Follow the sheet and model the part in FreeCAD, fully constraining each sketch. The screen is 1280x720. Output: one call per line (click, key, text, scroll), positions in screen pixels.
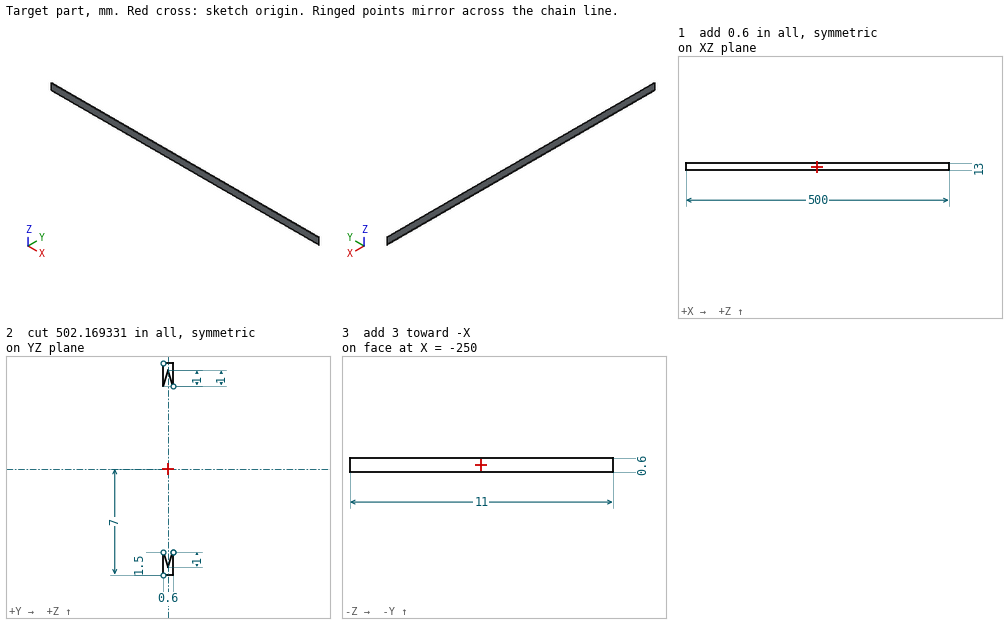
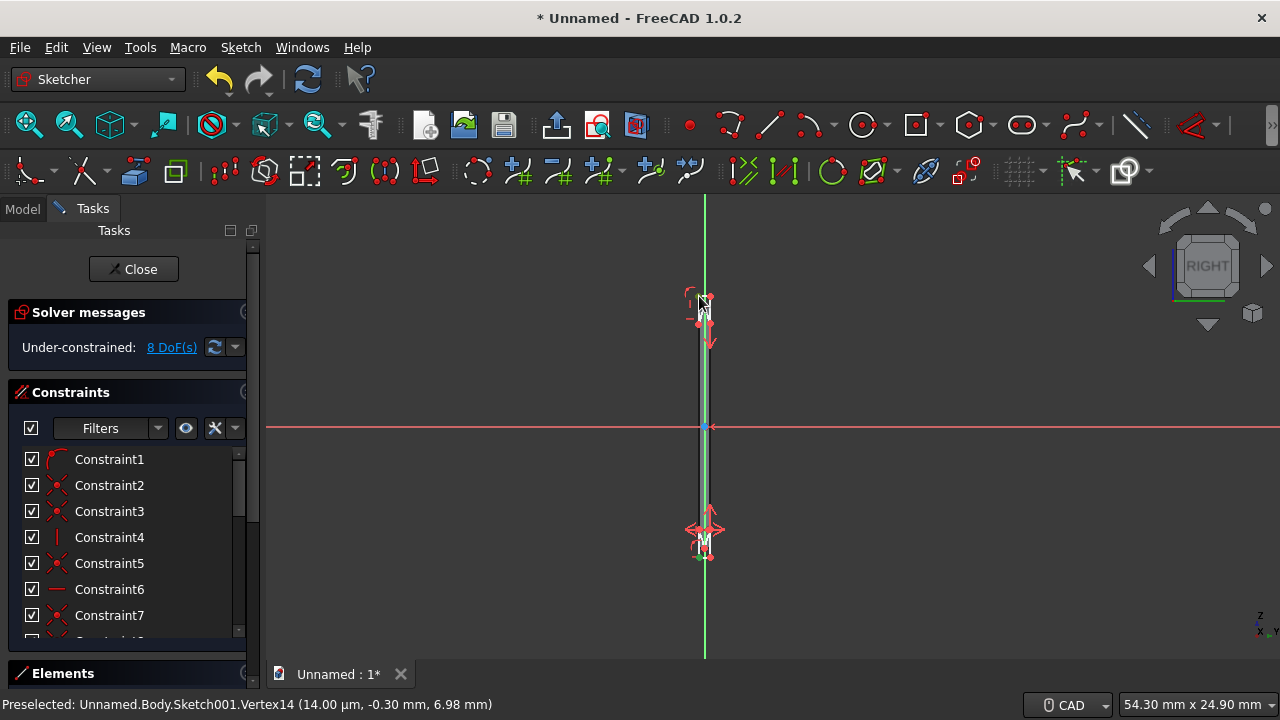
click(353, 426)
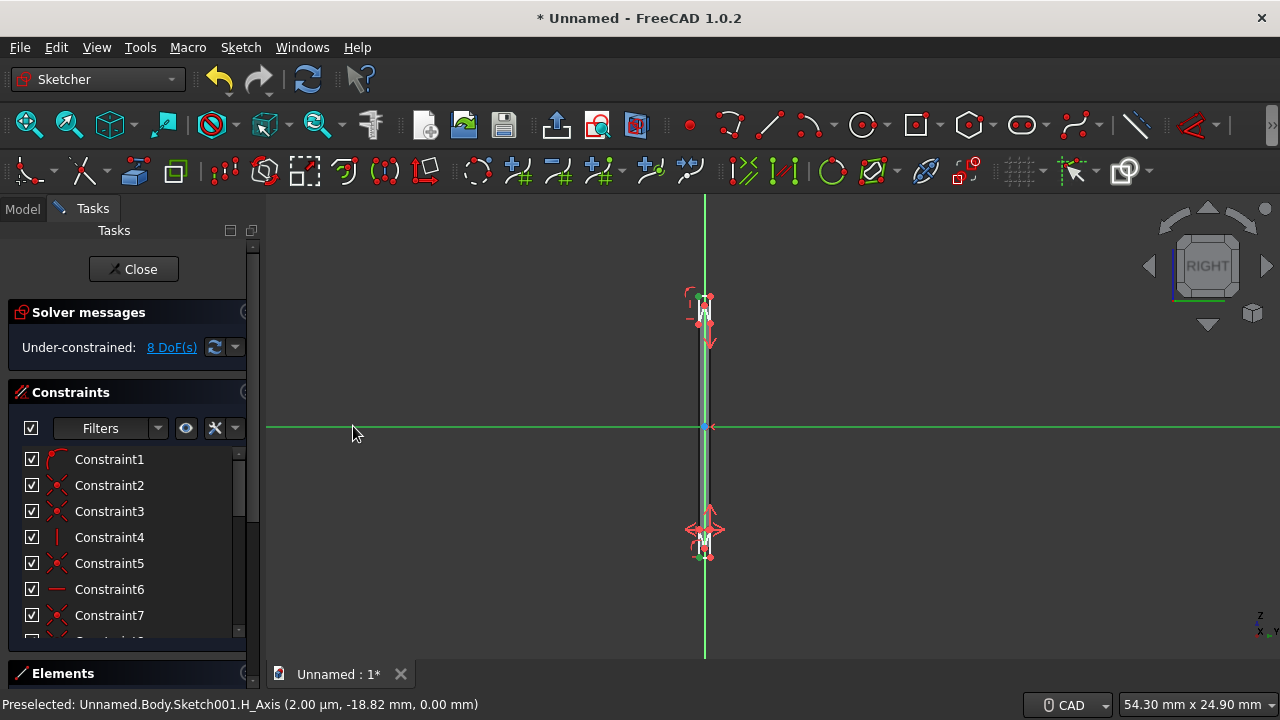
key(s)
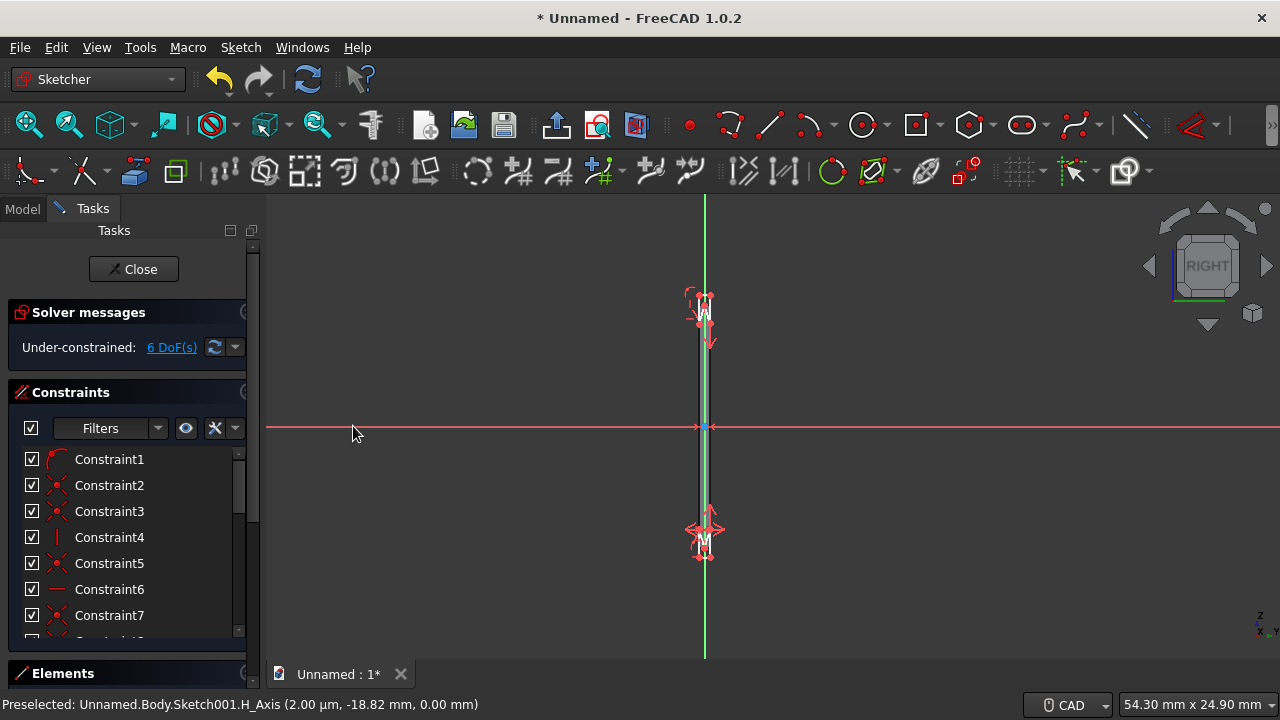
click(1192, 126)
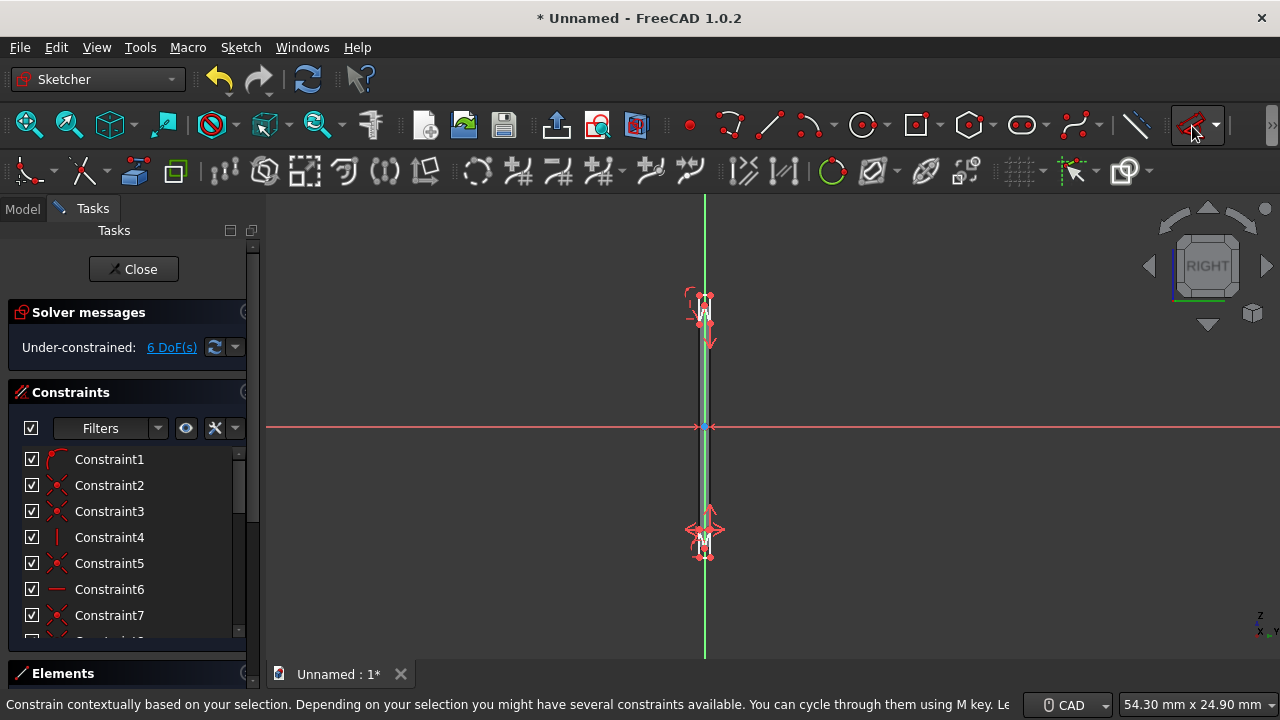
click(699, 558)
click(665, 492)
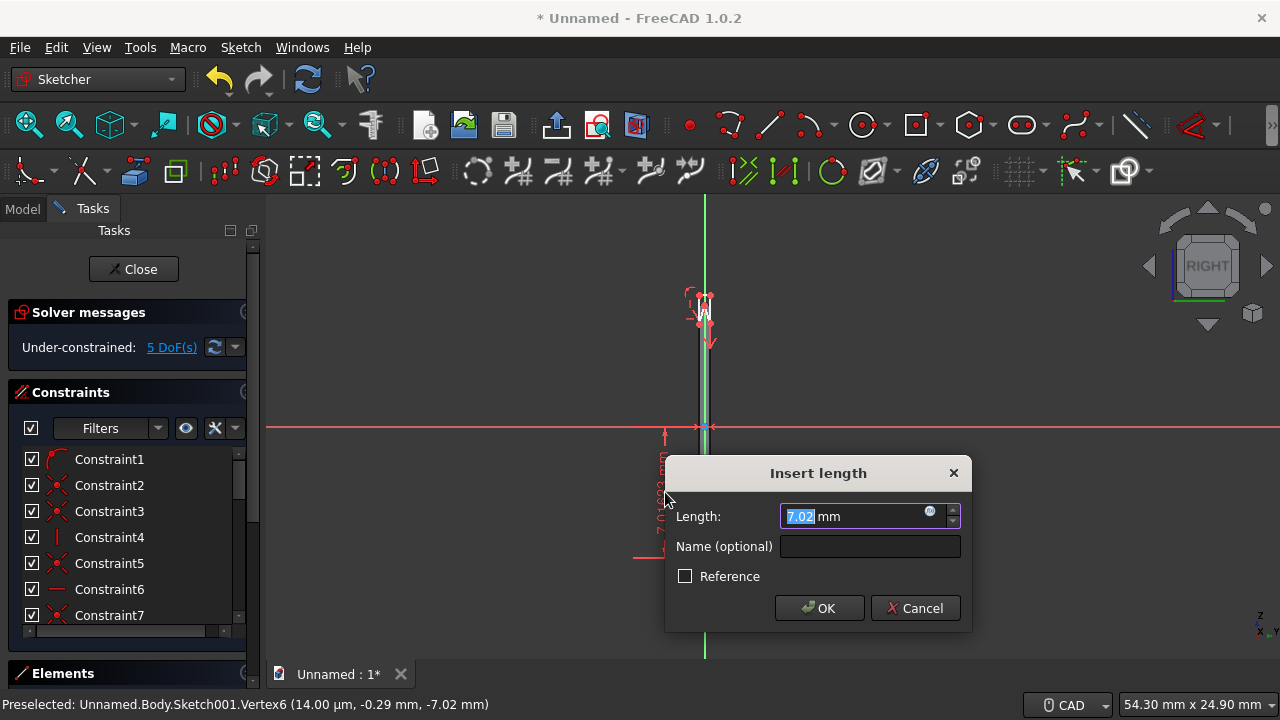
text(7)
key(Return)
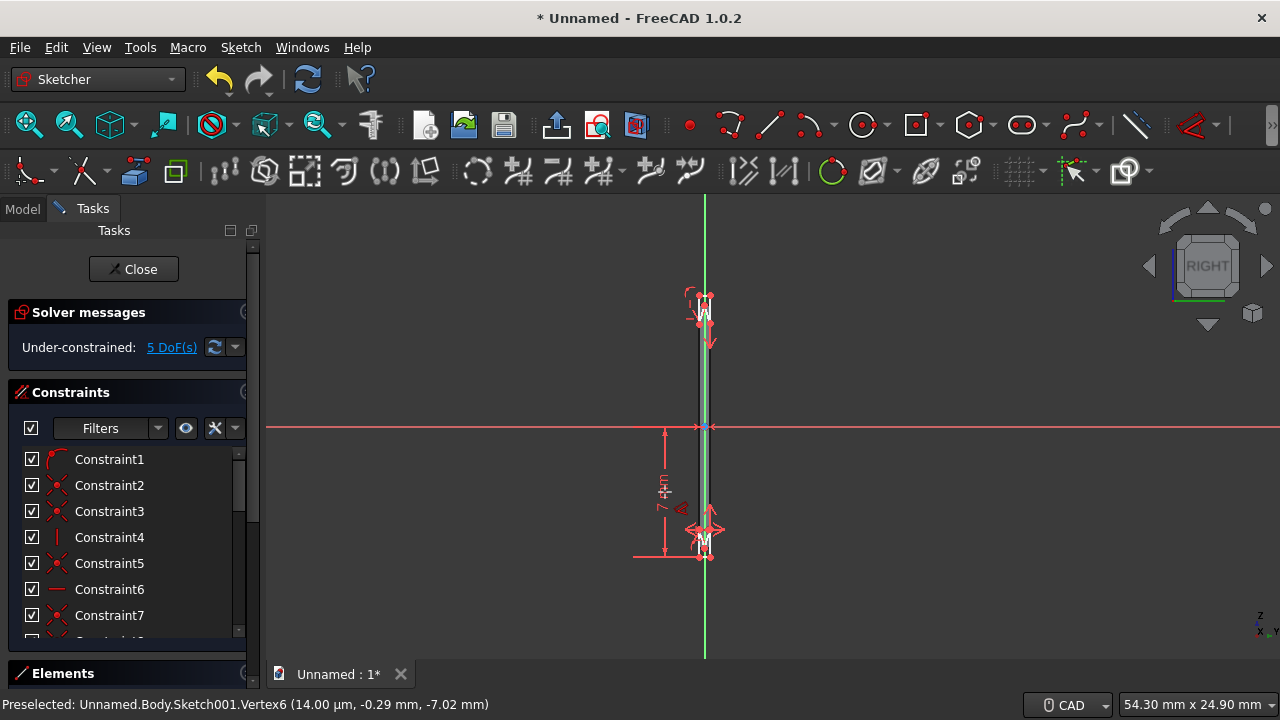
scroll(707, 541, up, 8)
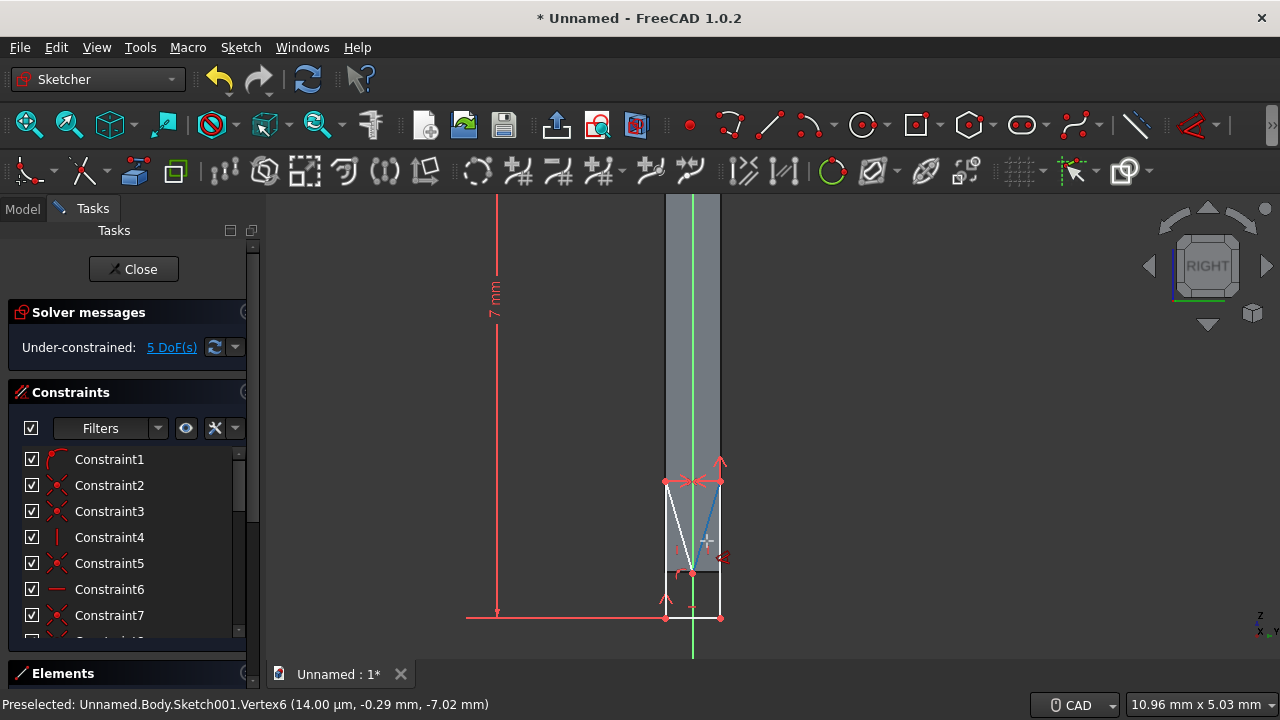
click(704, 537)
click(754, 527)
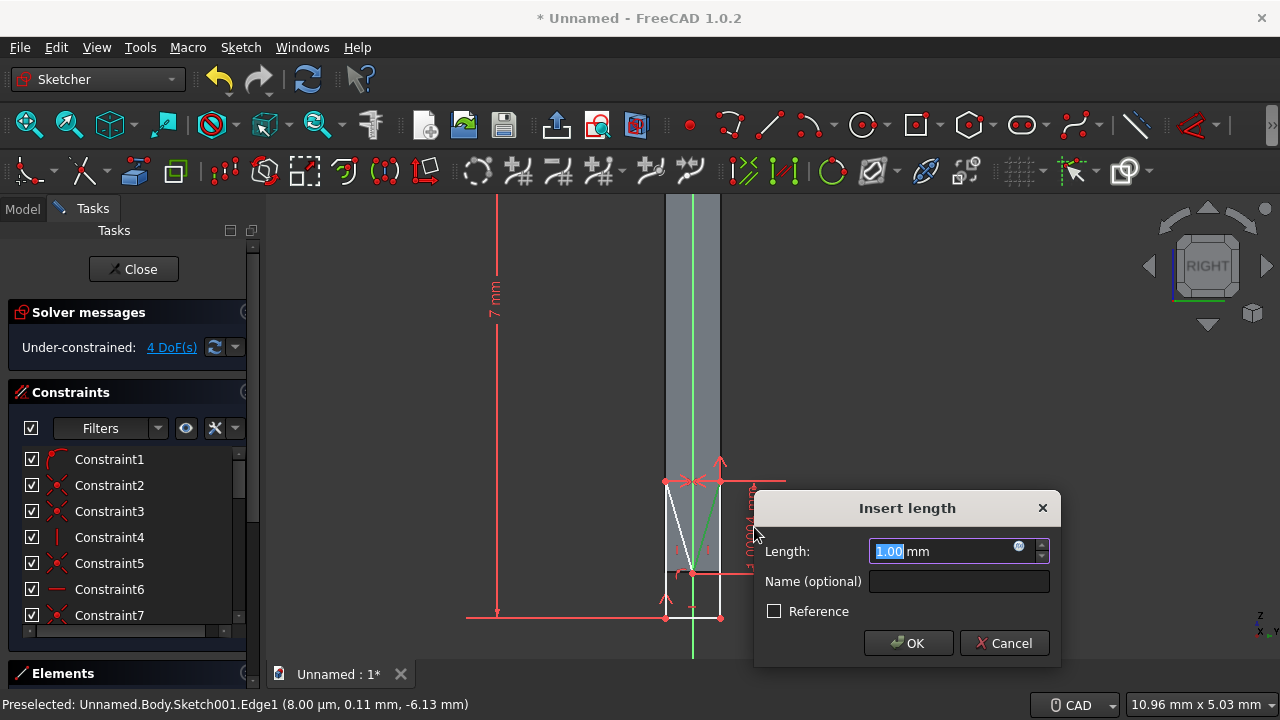
text(1)
key(Return)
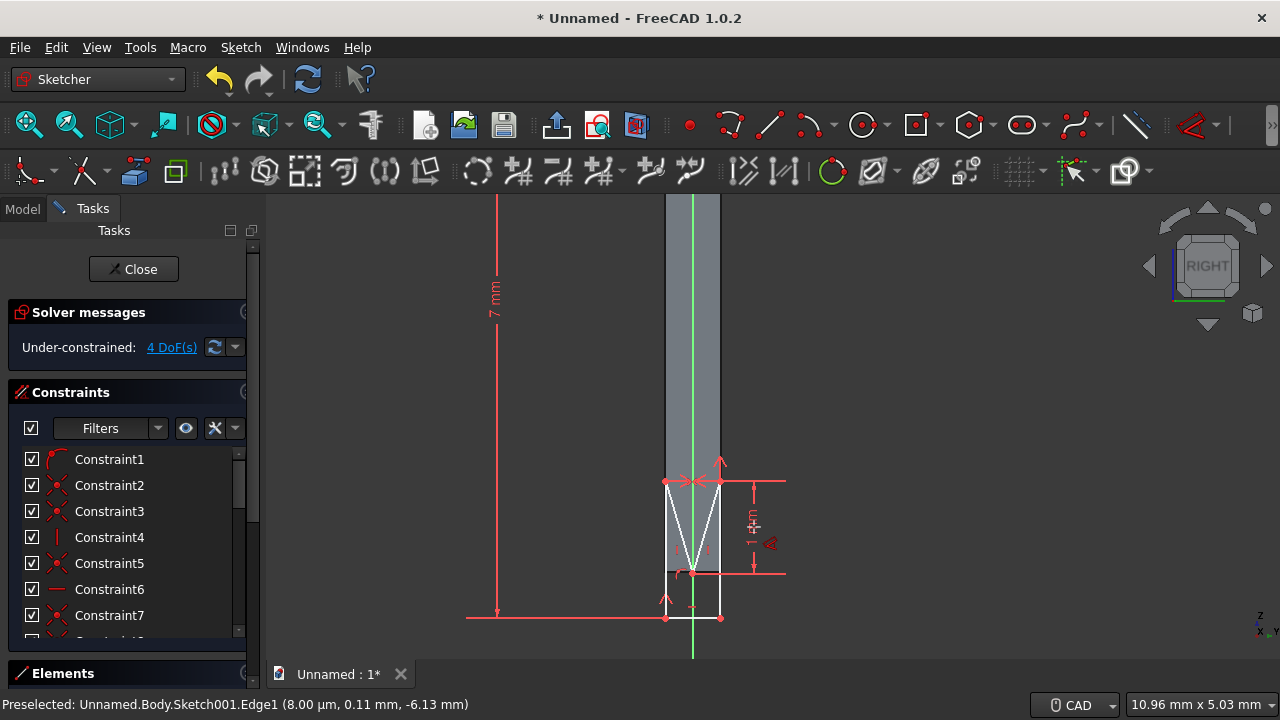
scroll(707, 542, down, 8)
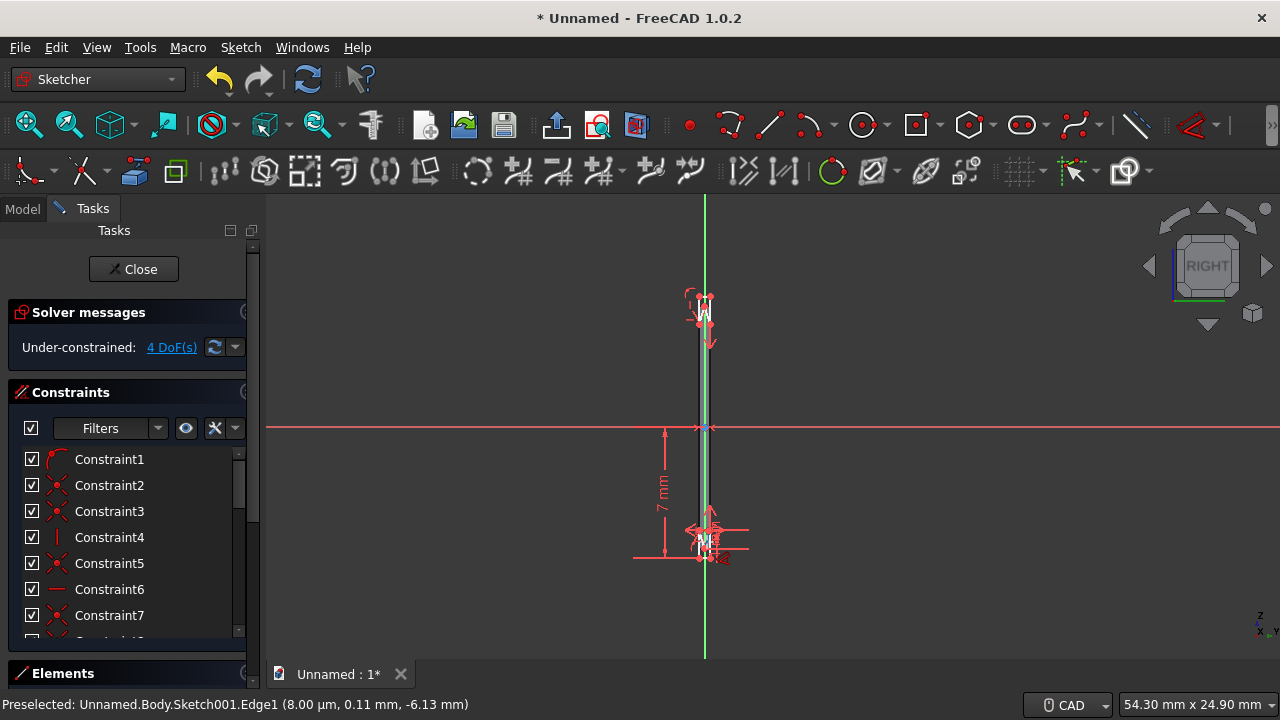
scroll(701, 317, up, 10)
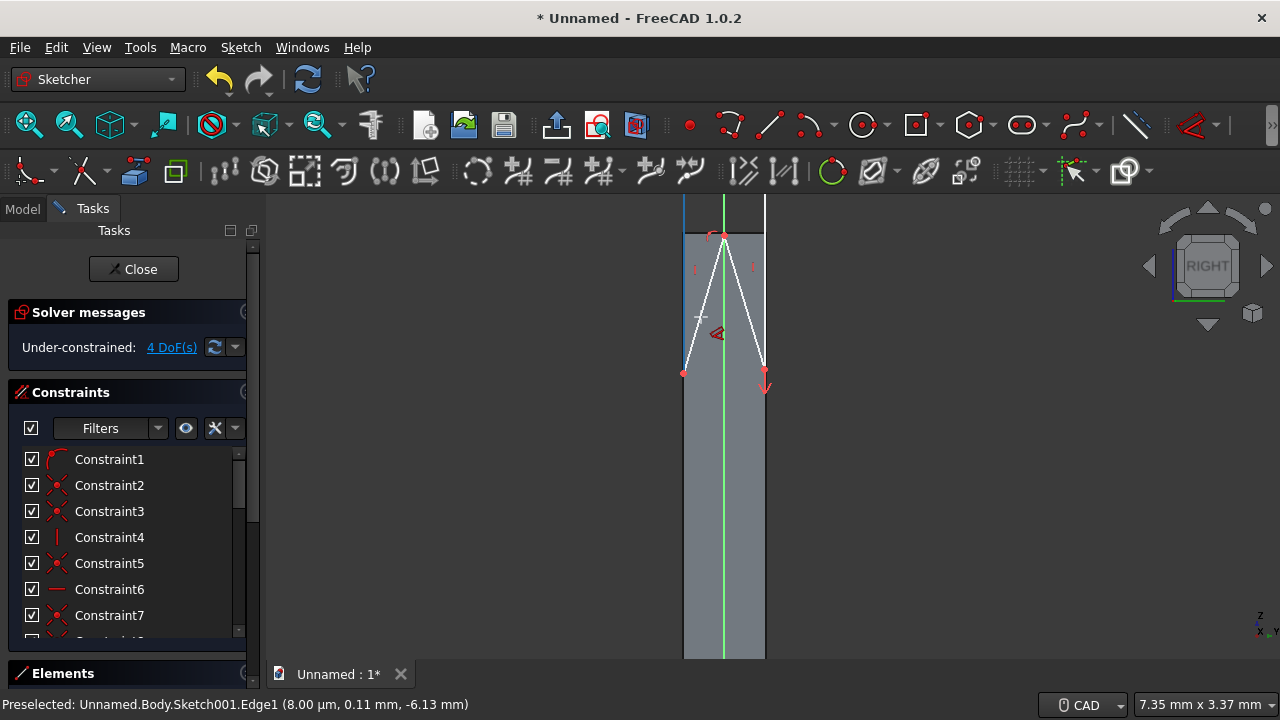
click(700, 318)
click(650, 305)